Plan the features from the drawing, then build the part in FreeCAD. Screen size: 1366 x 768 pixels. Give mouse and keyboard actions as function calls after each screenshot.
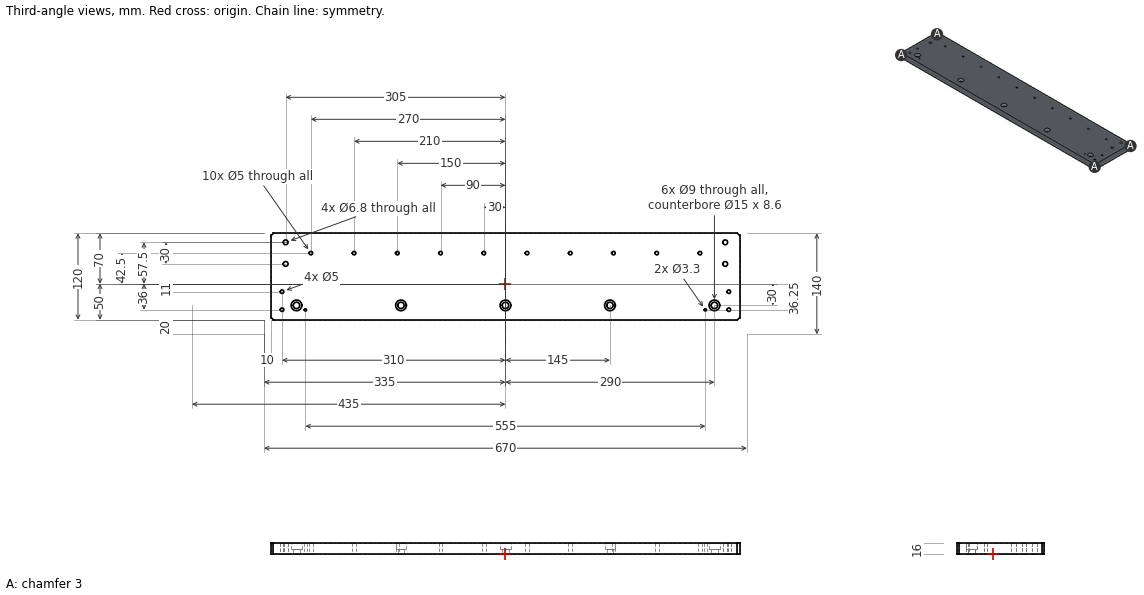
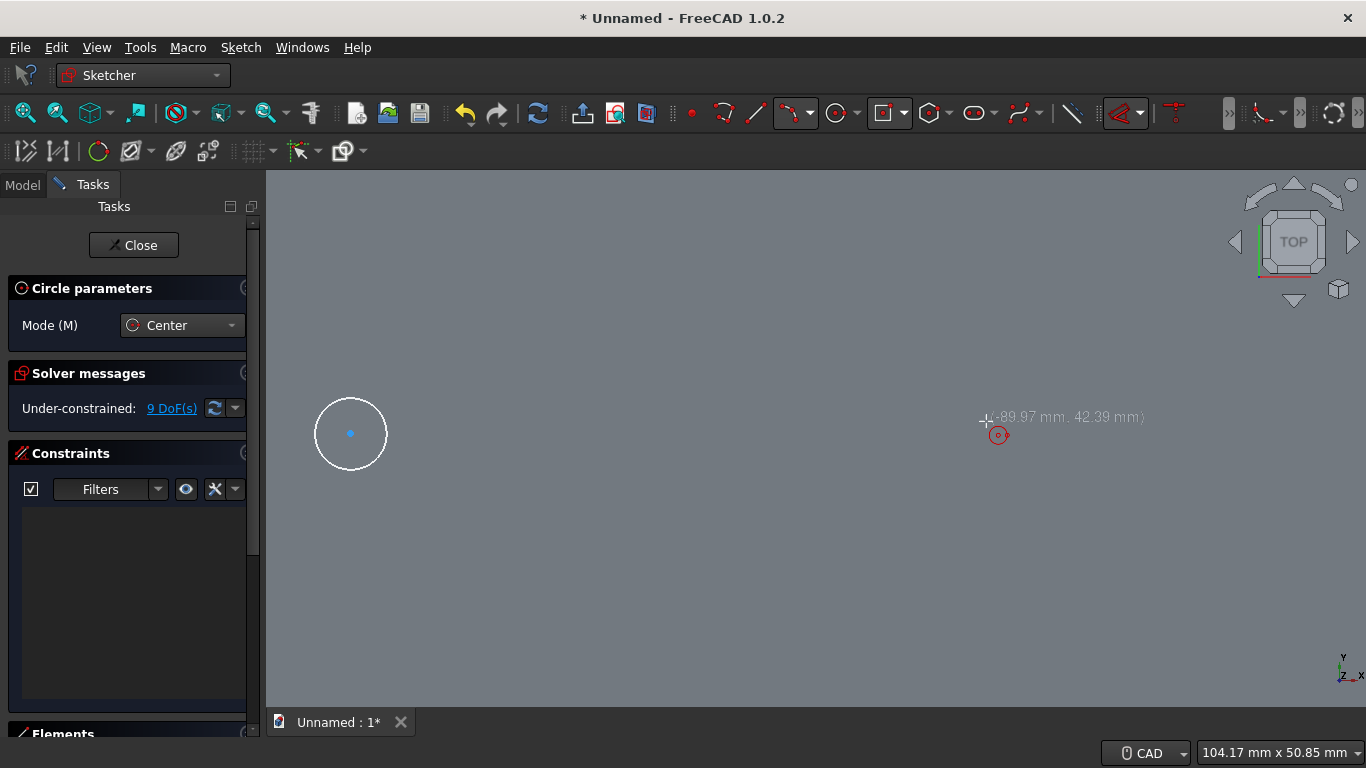
scroll(599, 414, down, 11)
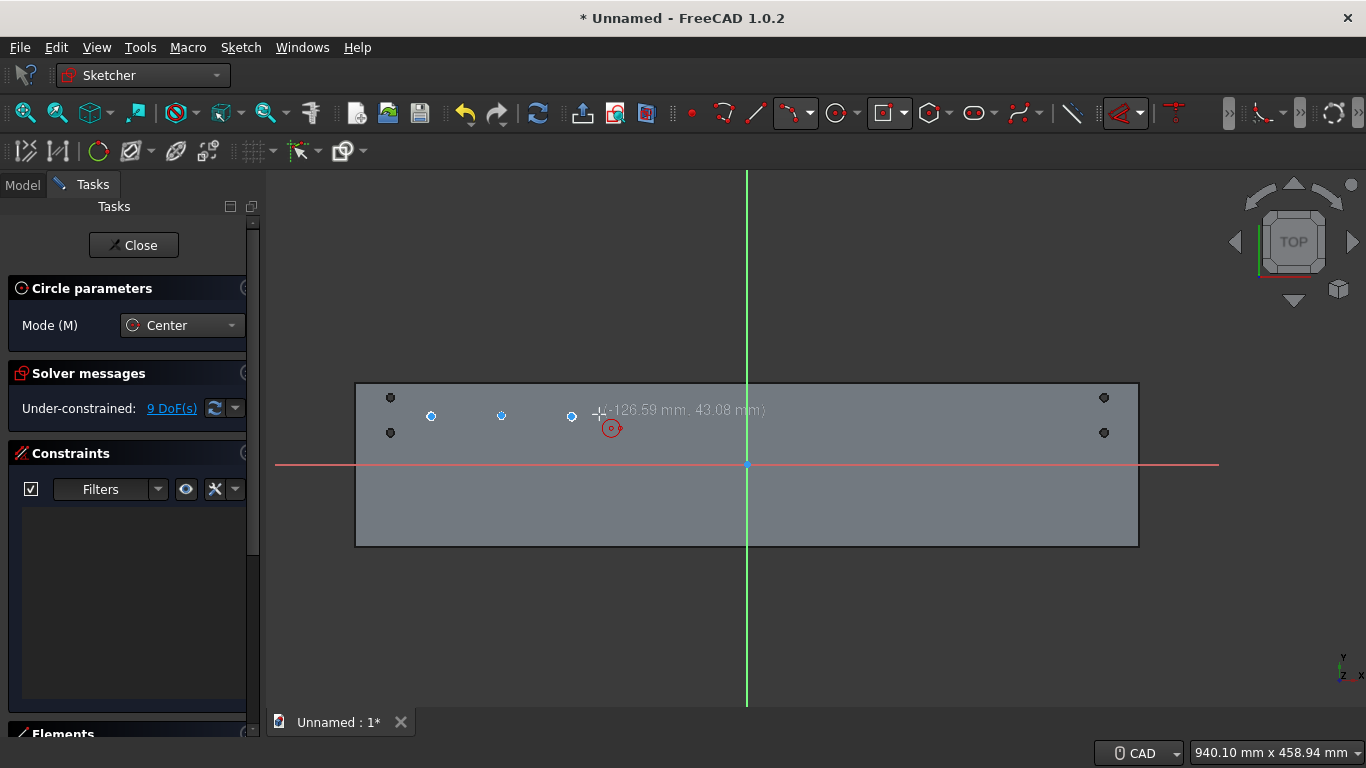
click(642, 415)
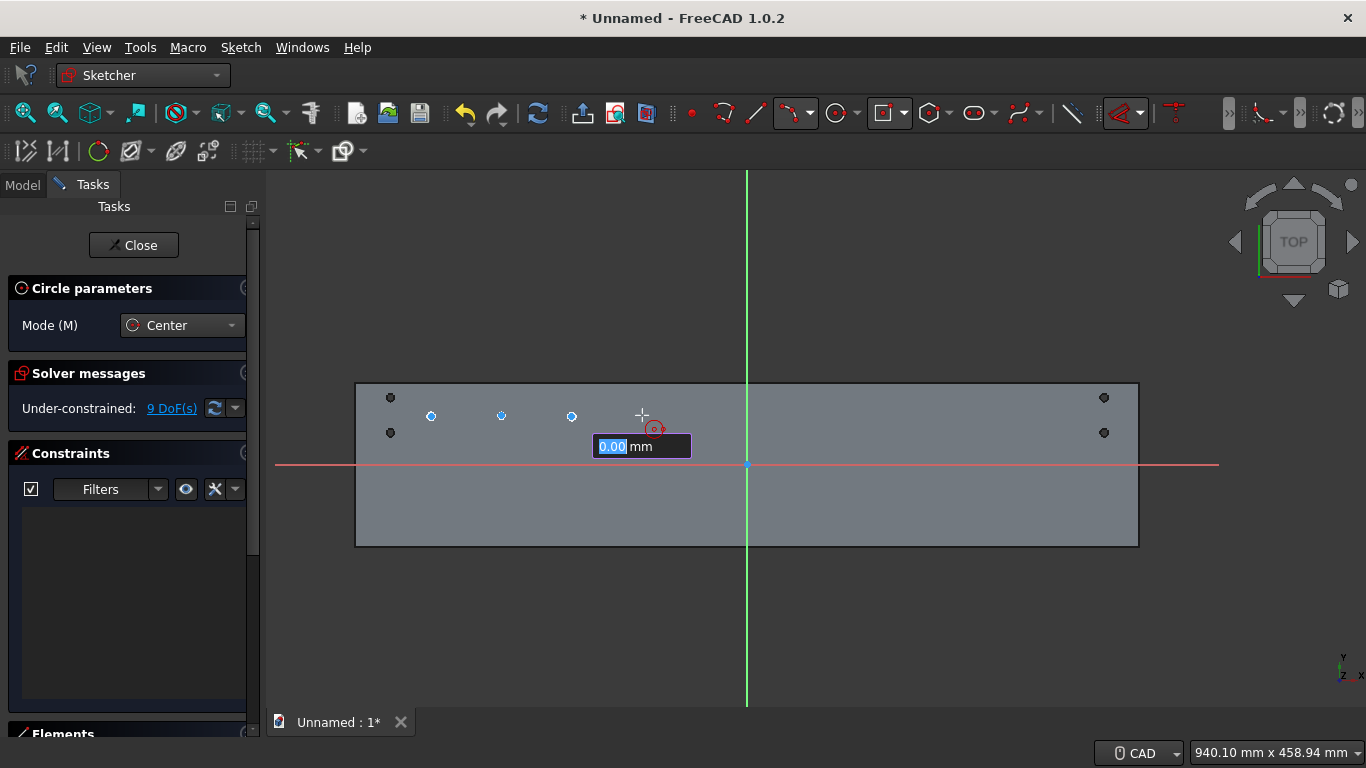
scroll(644, 413, up, 9)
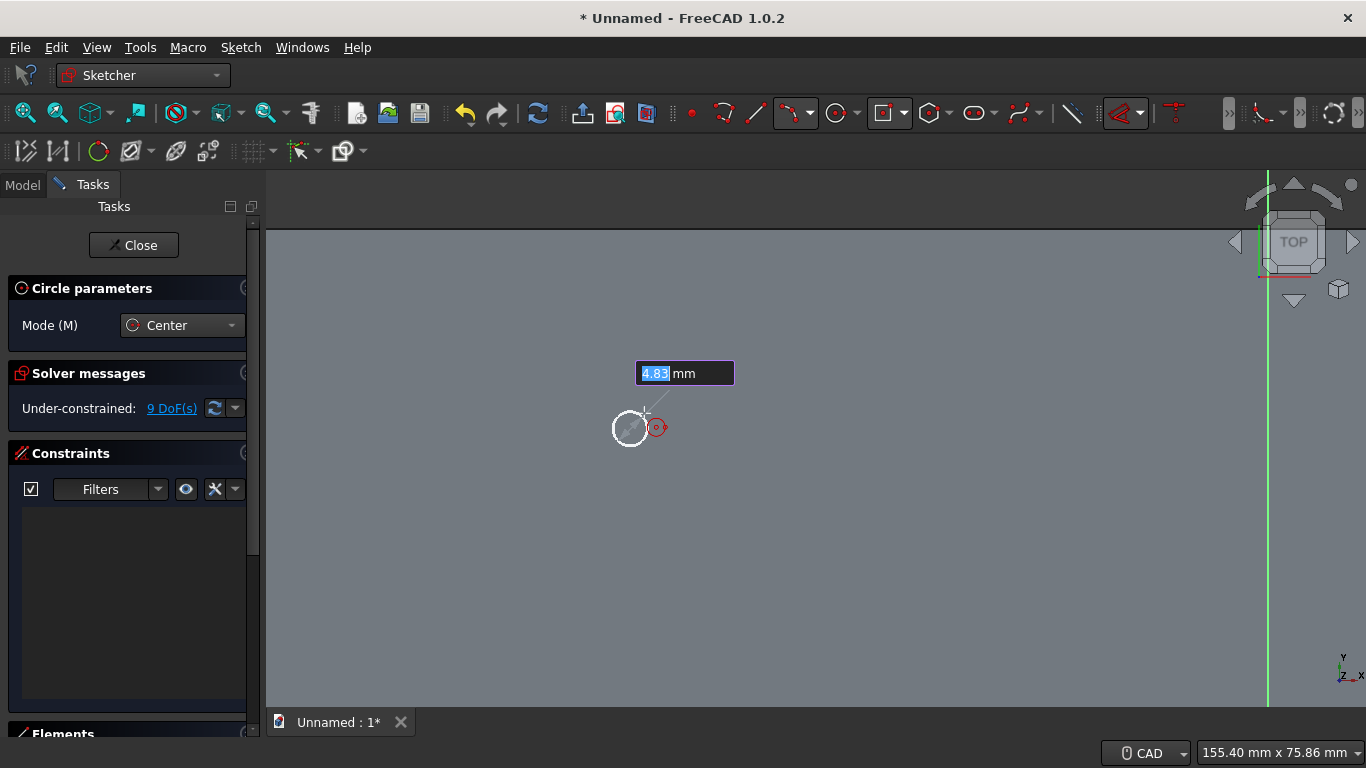
click(643, 411)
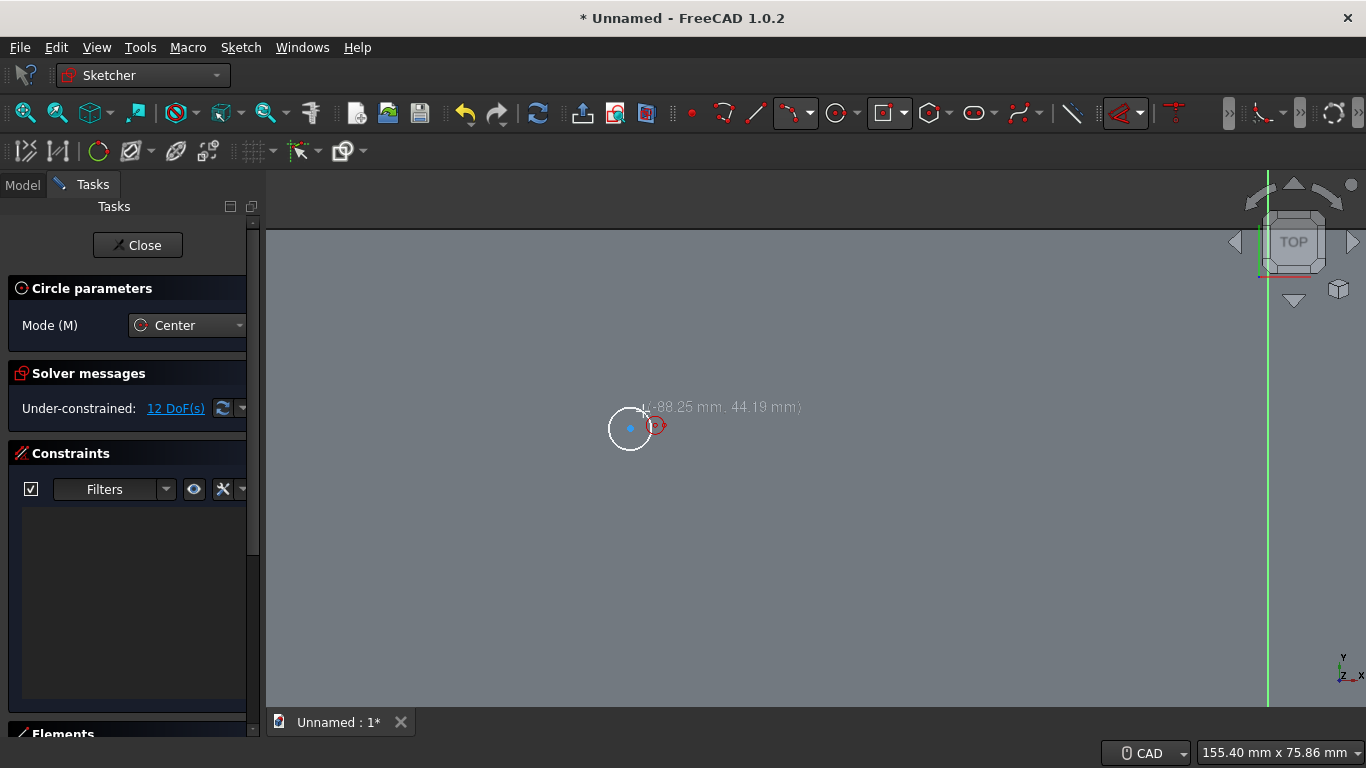
scroll(1055, 424, up, 2)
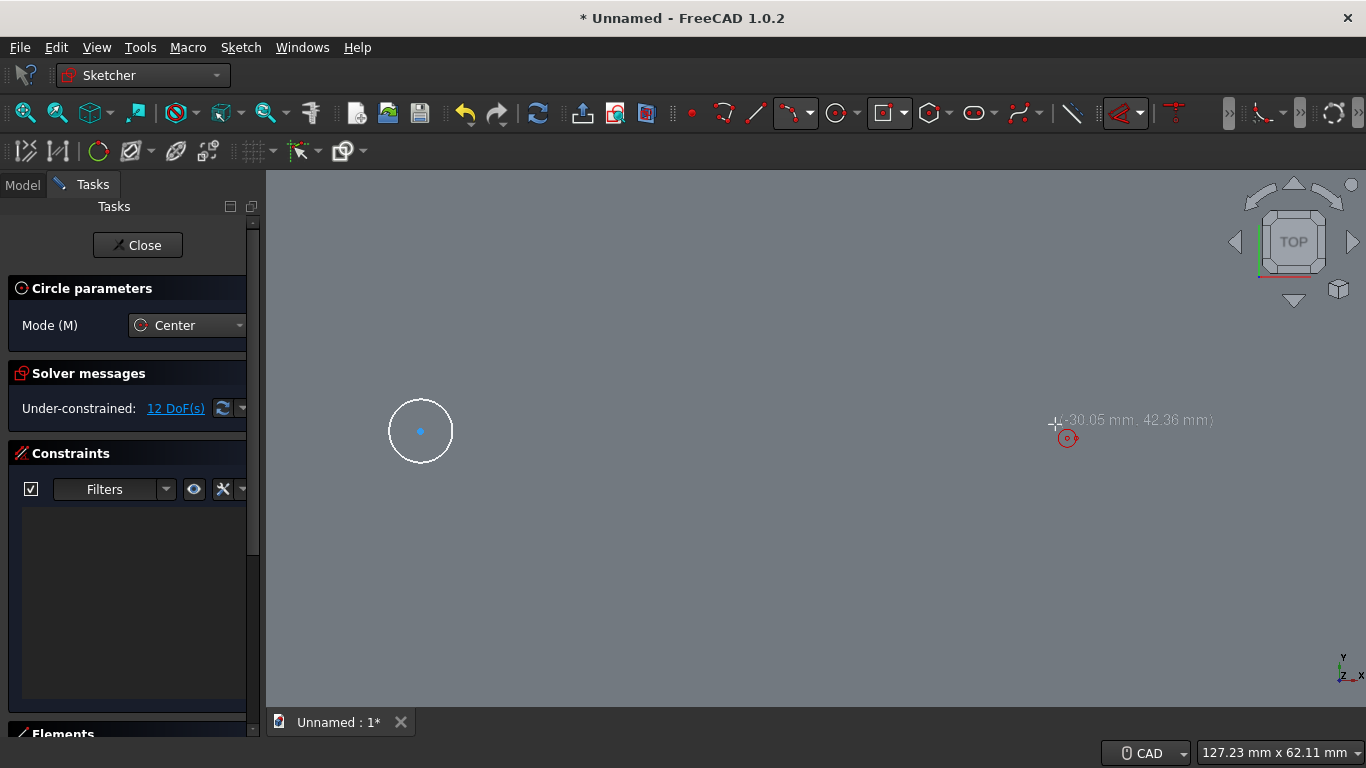
scroll(670, 414, down, 11)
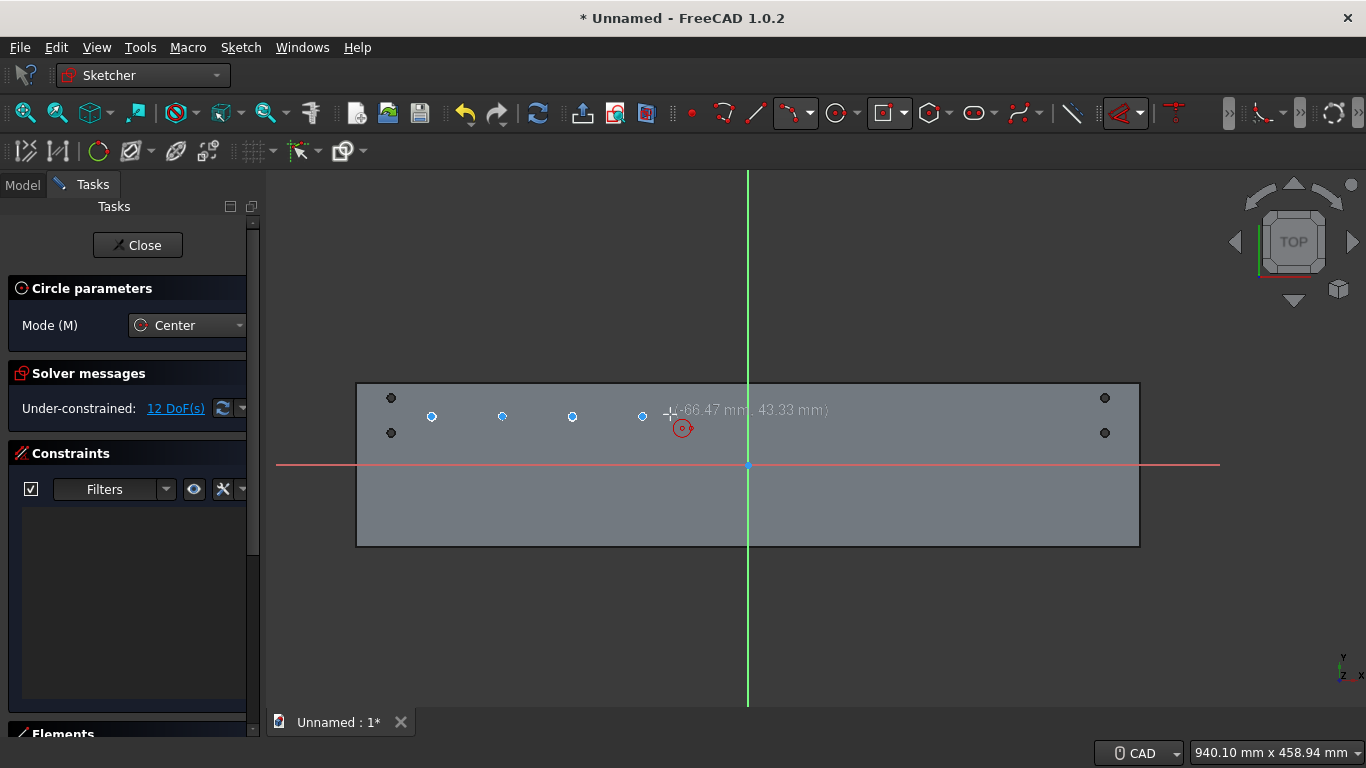
click(713, 415)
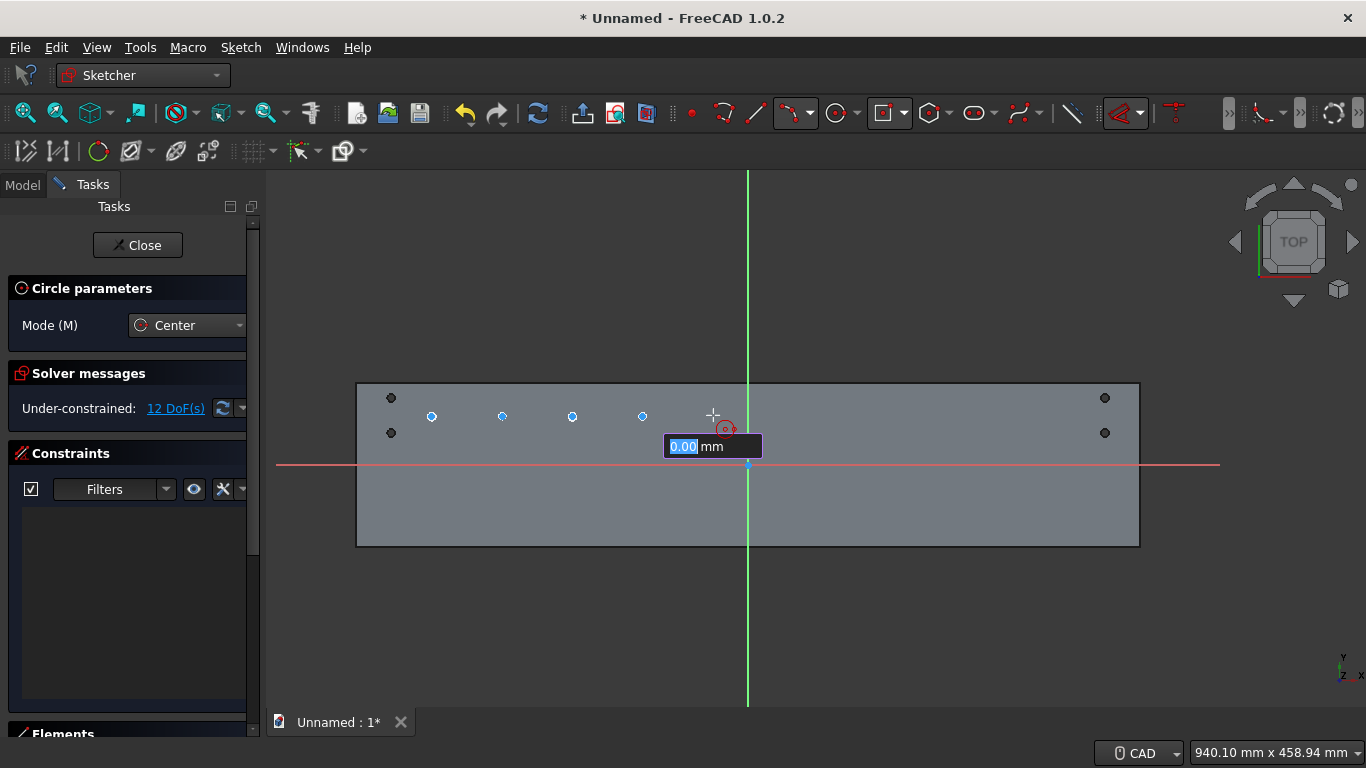
scroll(715, 413, up, 9)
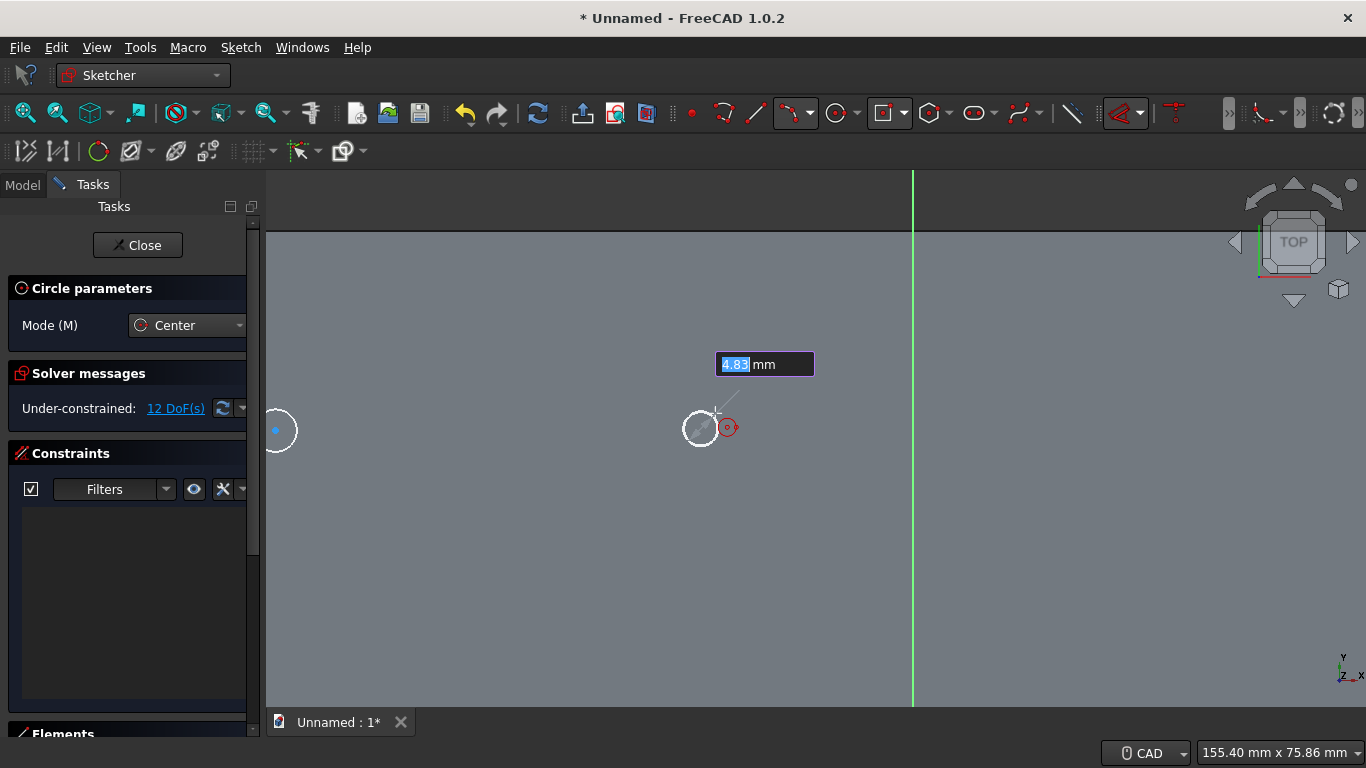
click(713, 413)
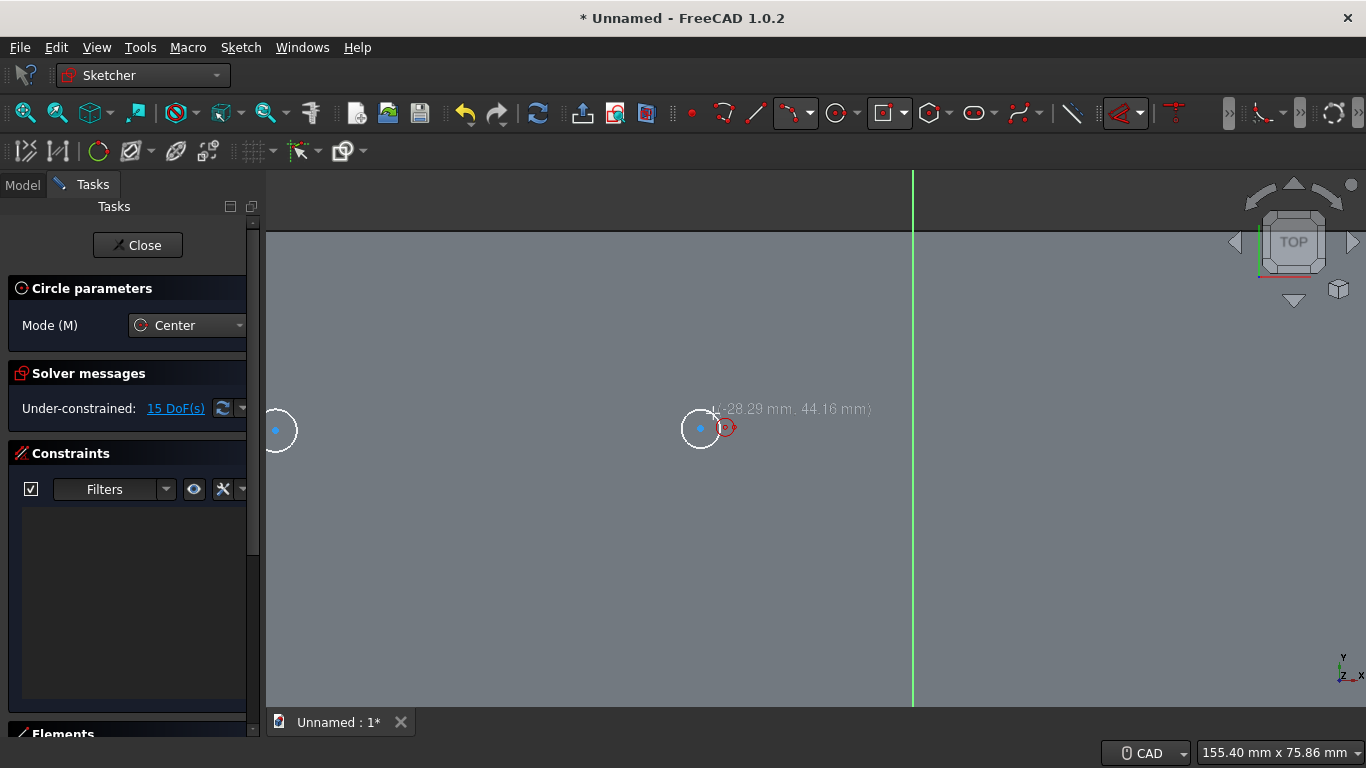
scroll(1126, 426, up, 2)